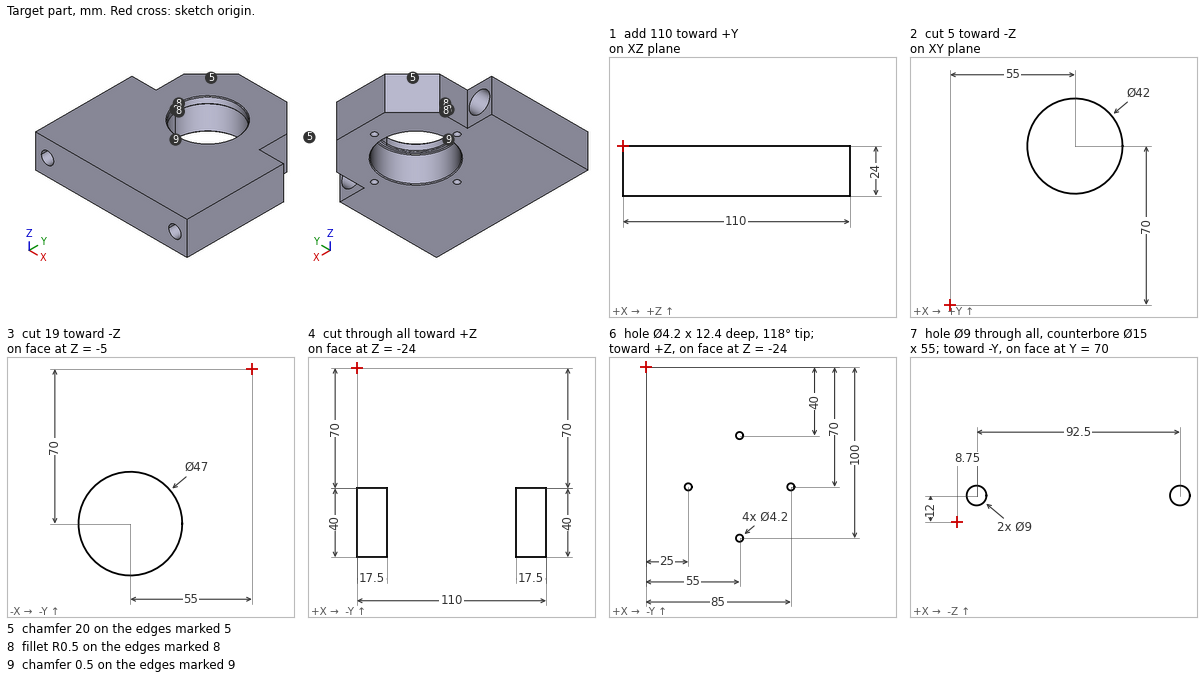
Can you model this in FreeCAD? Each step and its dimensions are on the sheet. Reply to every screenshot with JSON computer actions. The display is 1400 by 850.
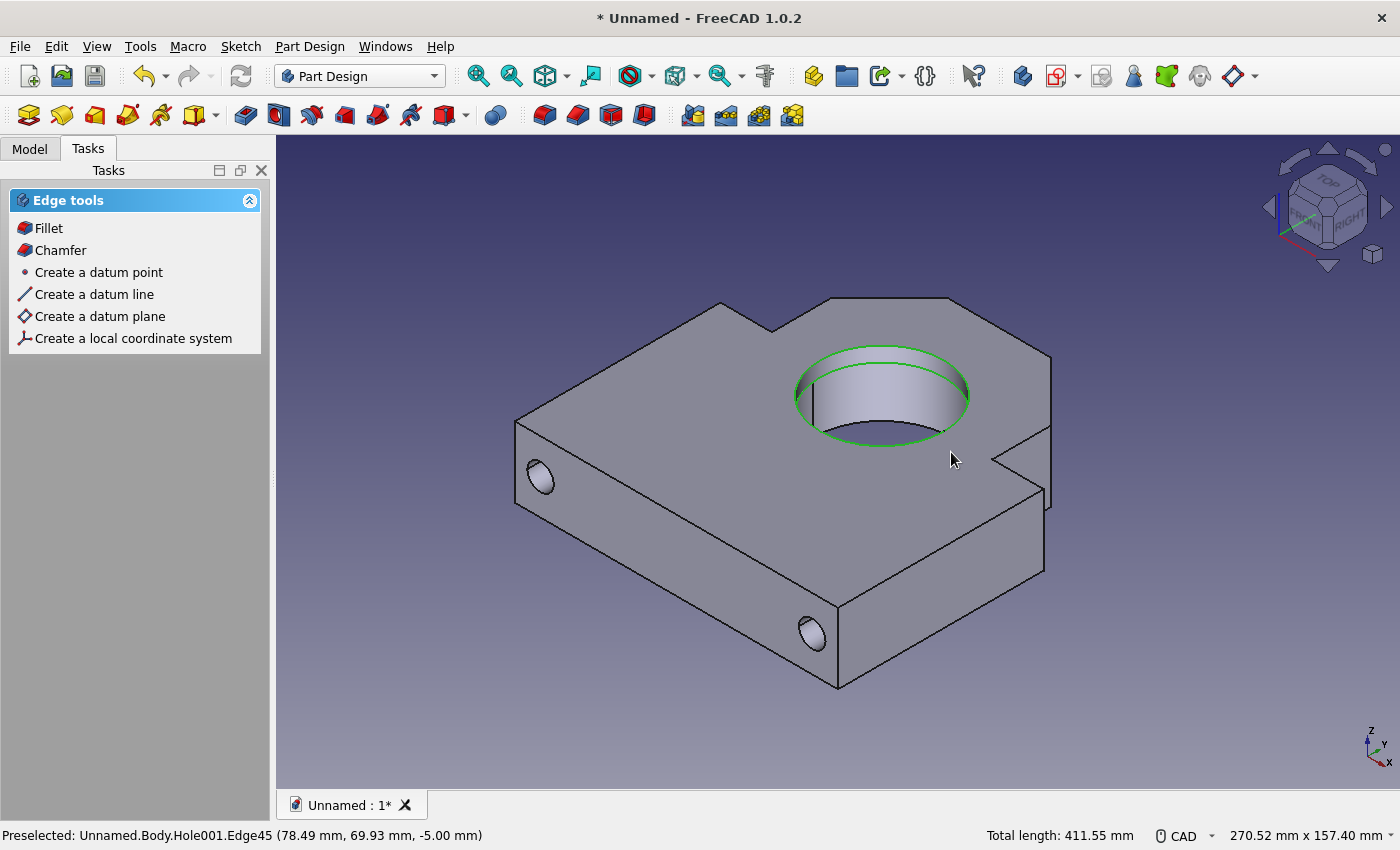
{"action": "left_click", "coordinate": [545, 116]}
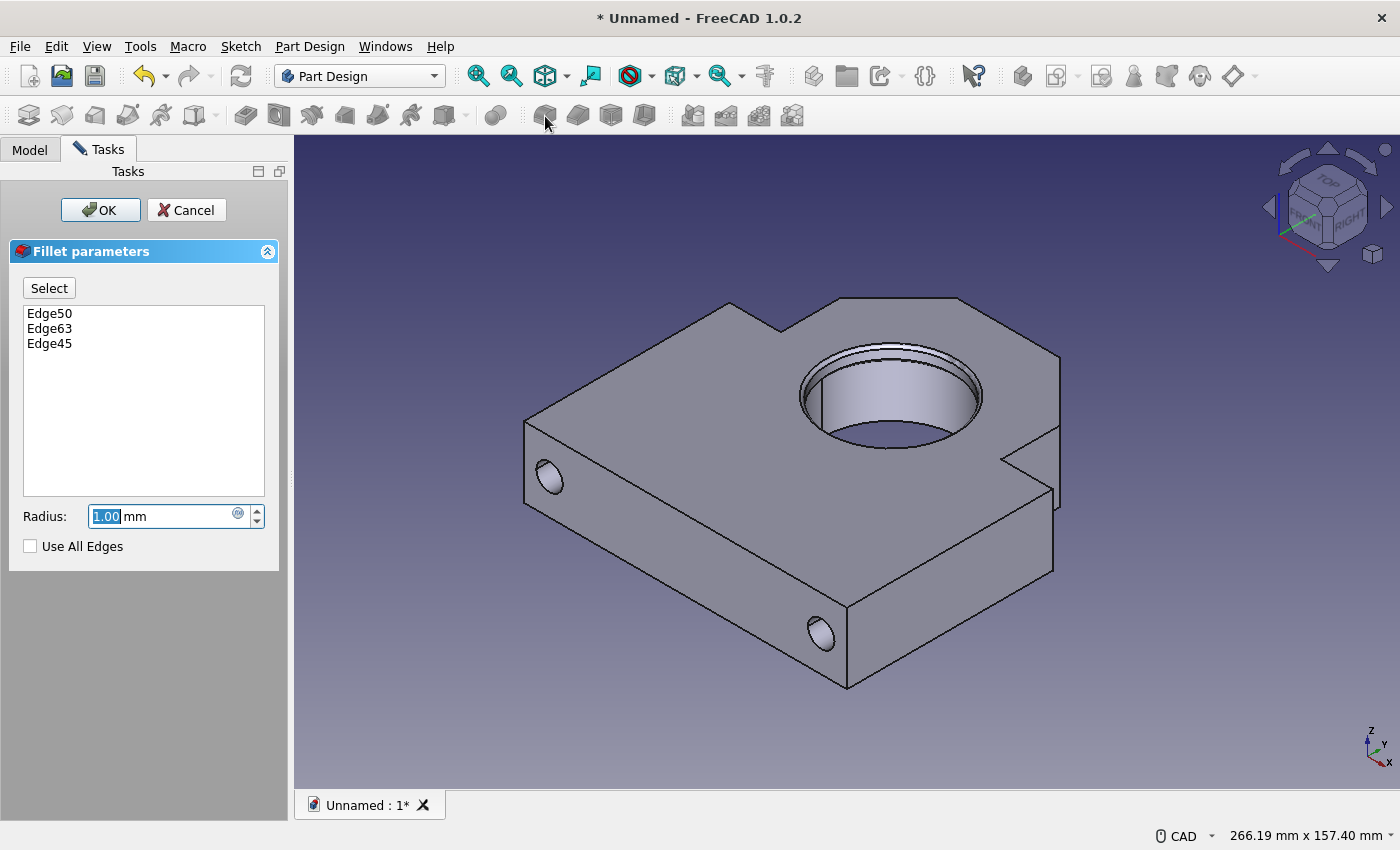
{"action": "type", "text": "0.5"}
{"action": "key", "text": "Tab"}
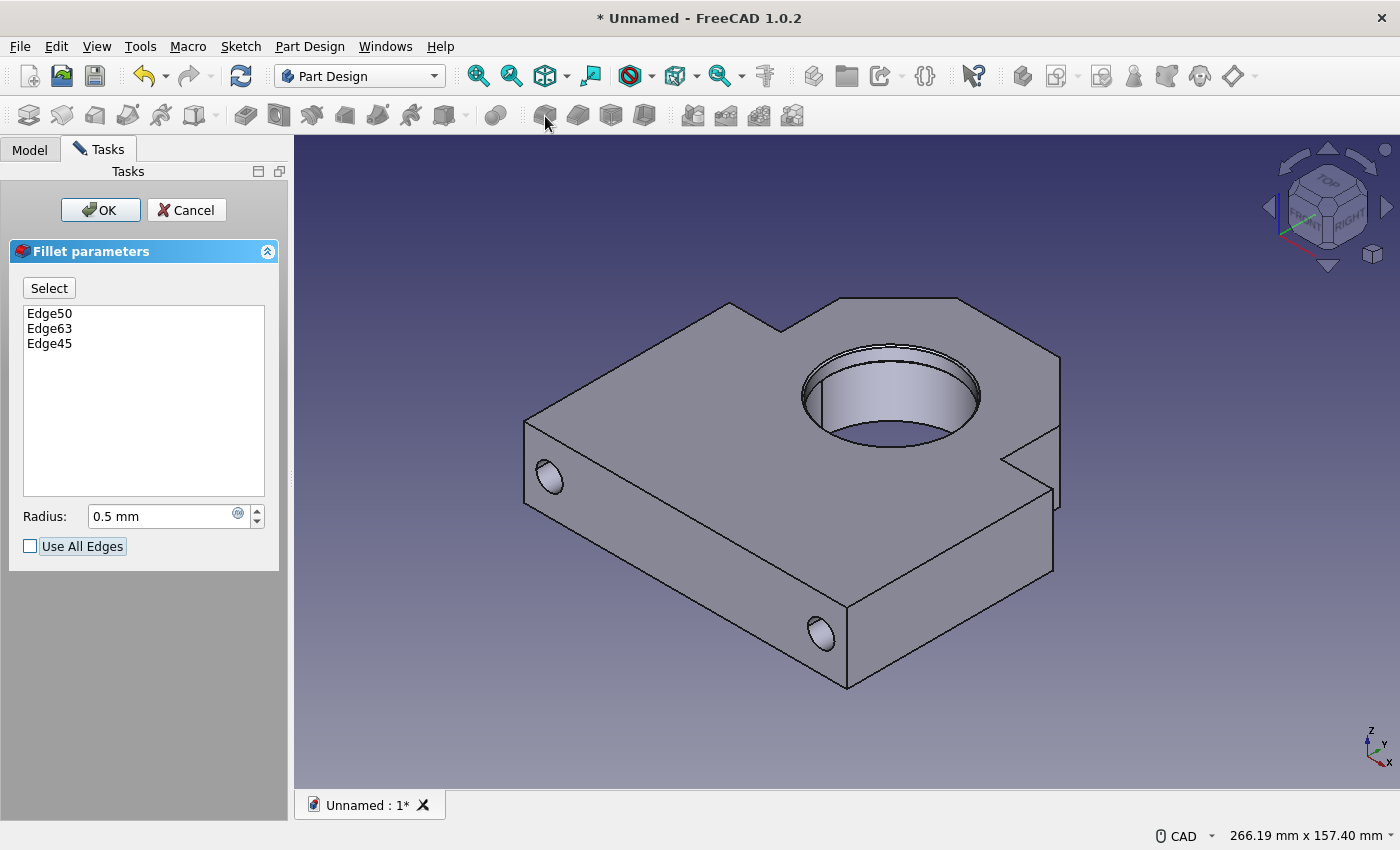
{"action": "left_click", "coordinate": [101, 210]}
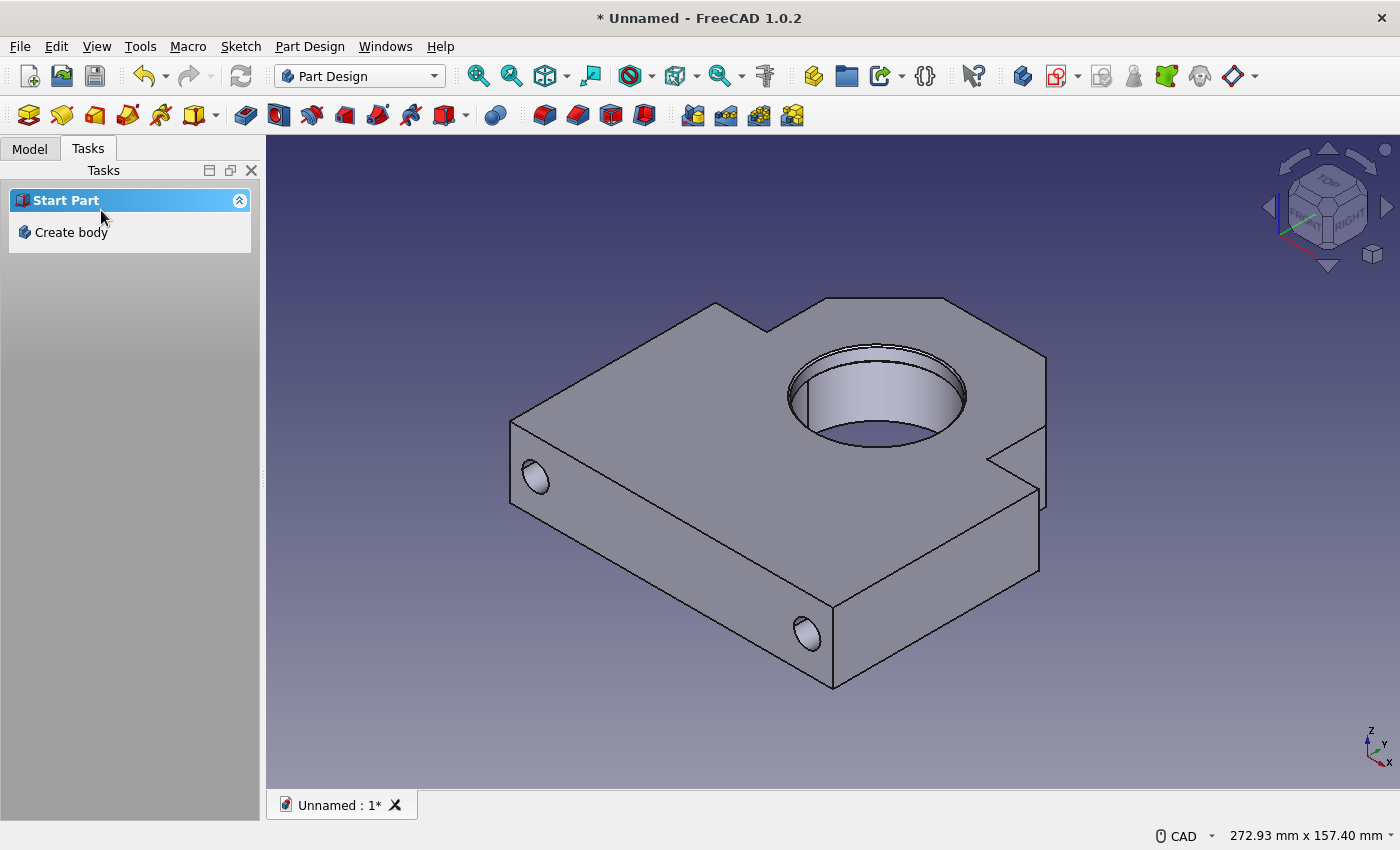
{"action": "key", "text": "2"}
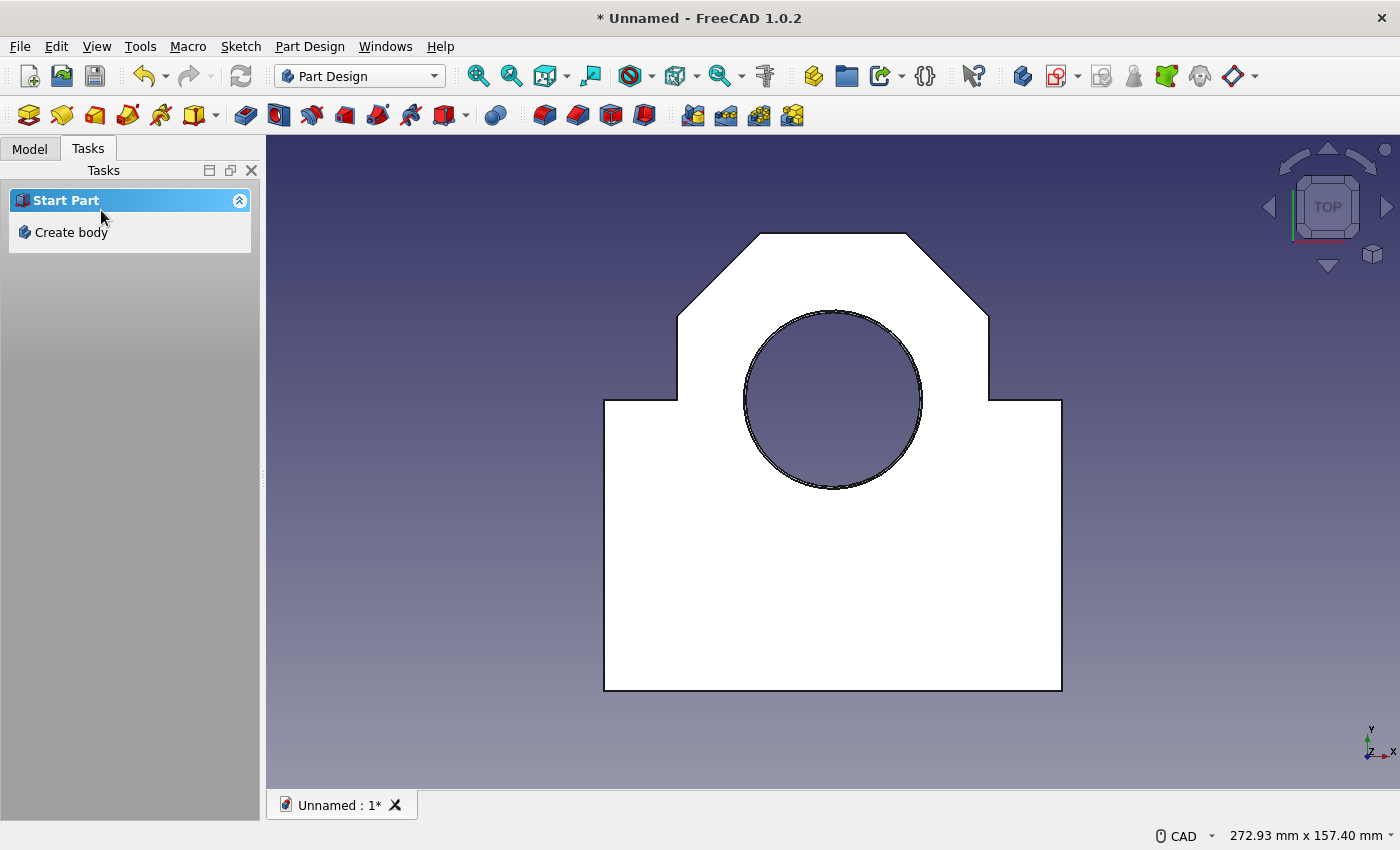
{"action": "key", "text": "0"}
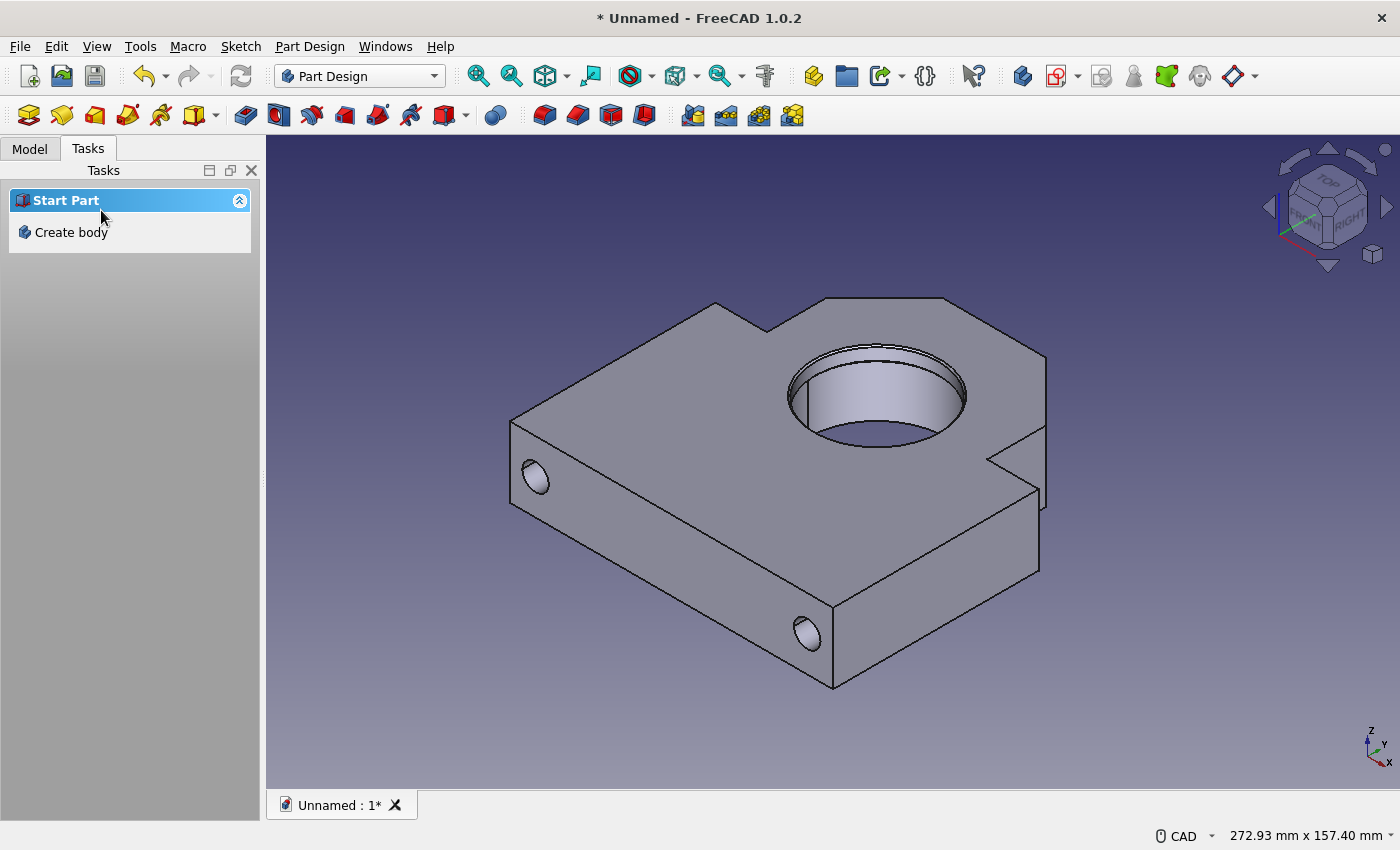
{"action": "key", "text": "1"}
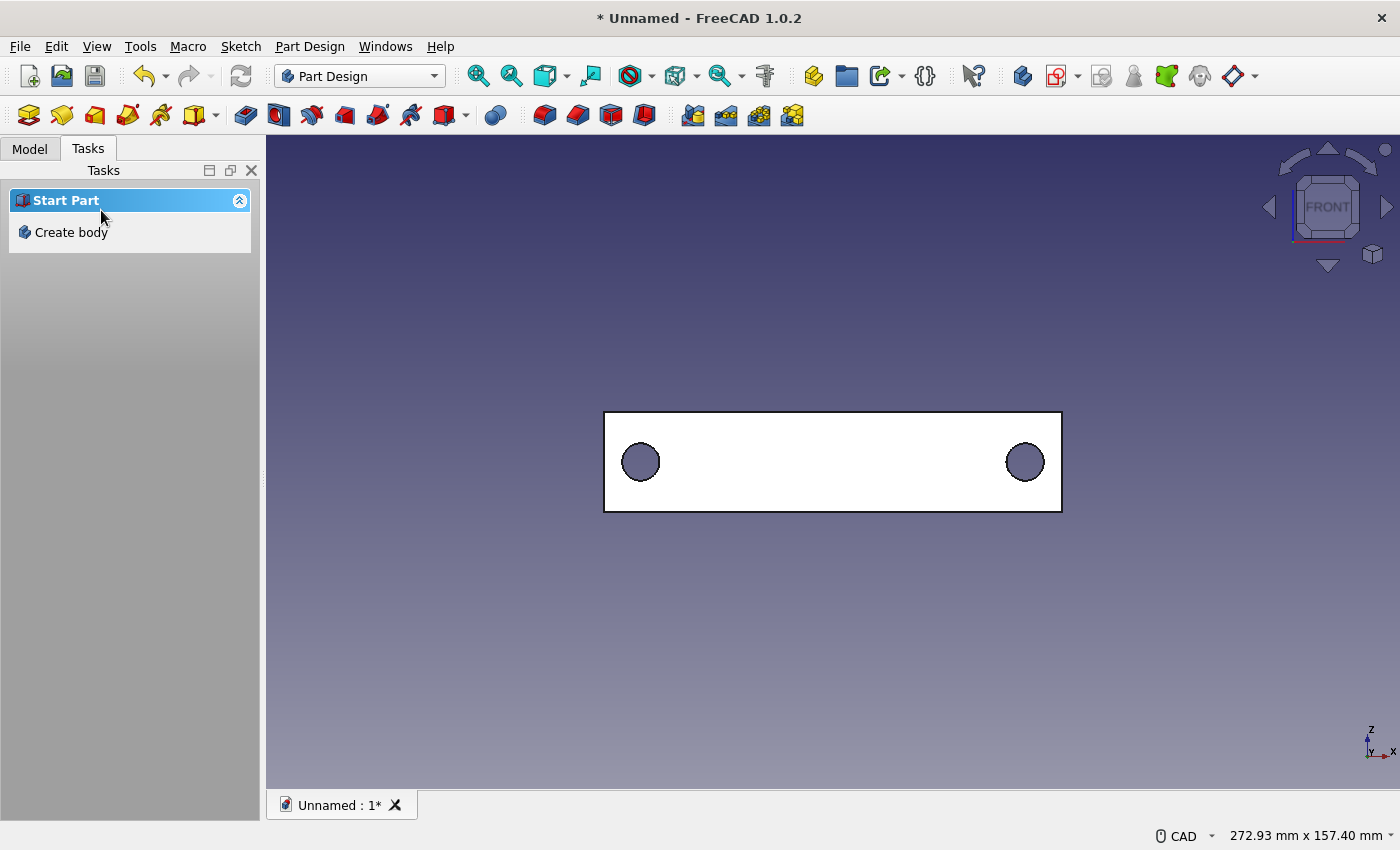
{"action": "left_click", "coordinate": [479, 76]}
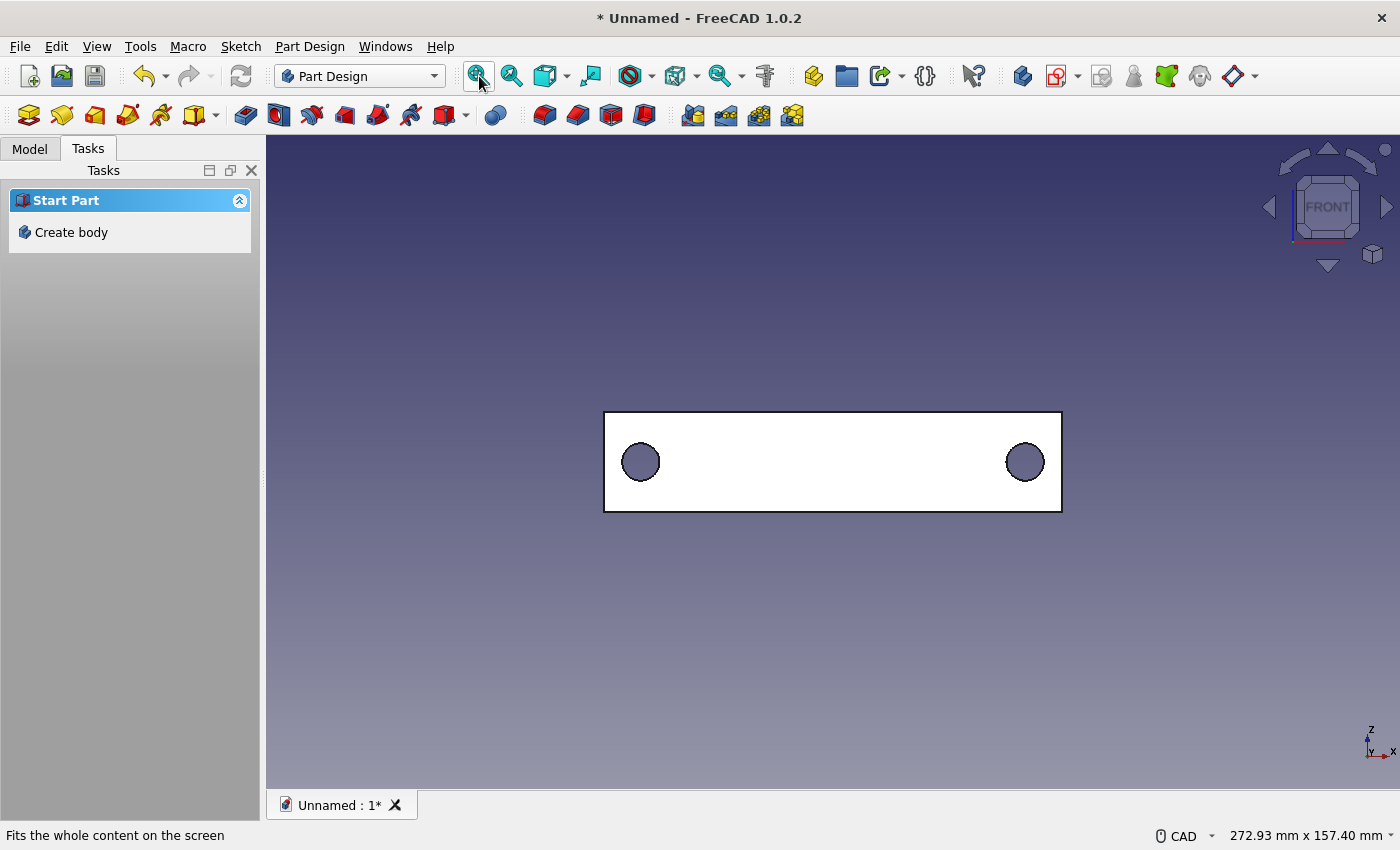
{"action": "key", "text": "3"}